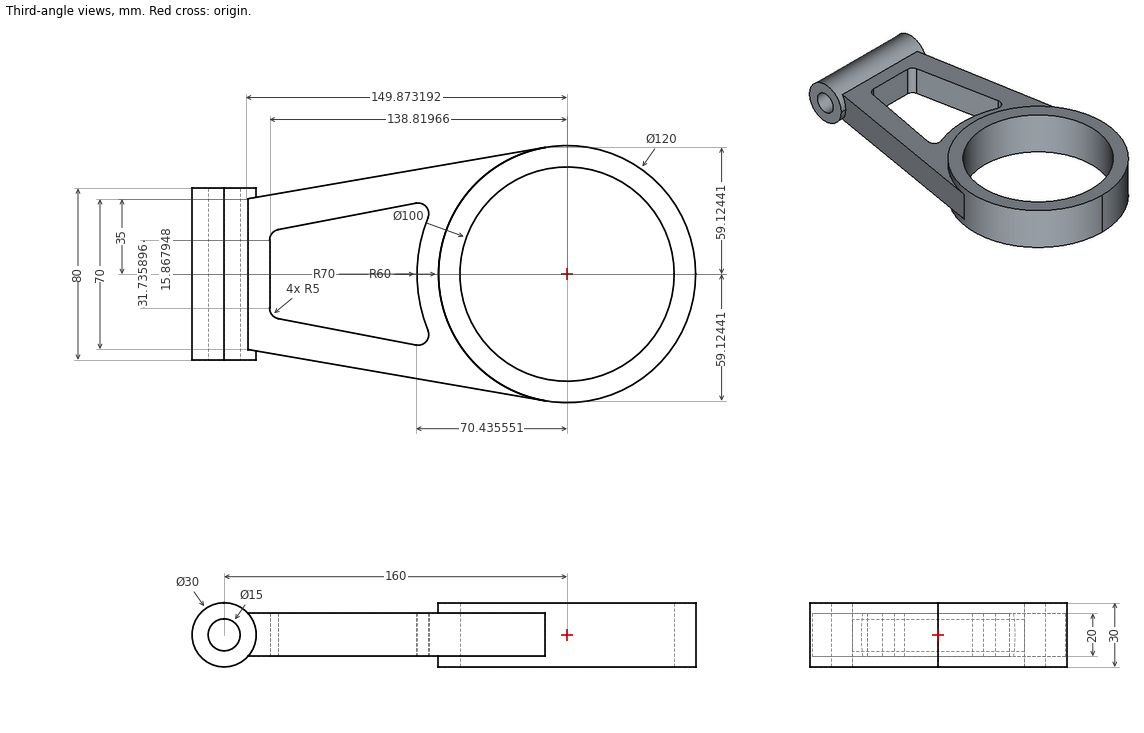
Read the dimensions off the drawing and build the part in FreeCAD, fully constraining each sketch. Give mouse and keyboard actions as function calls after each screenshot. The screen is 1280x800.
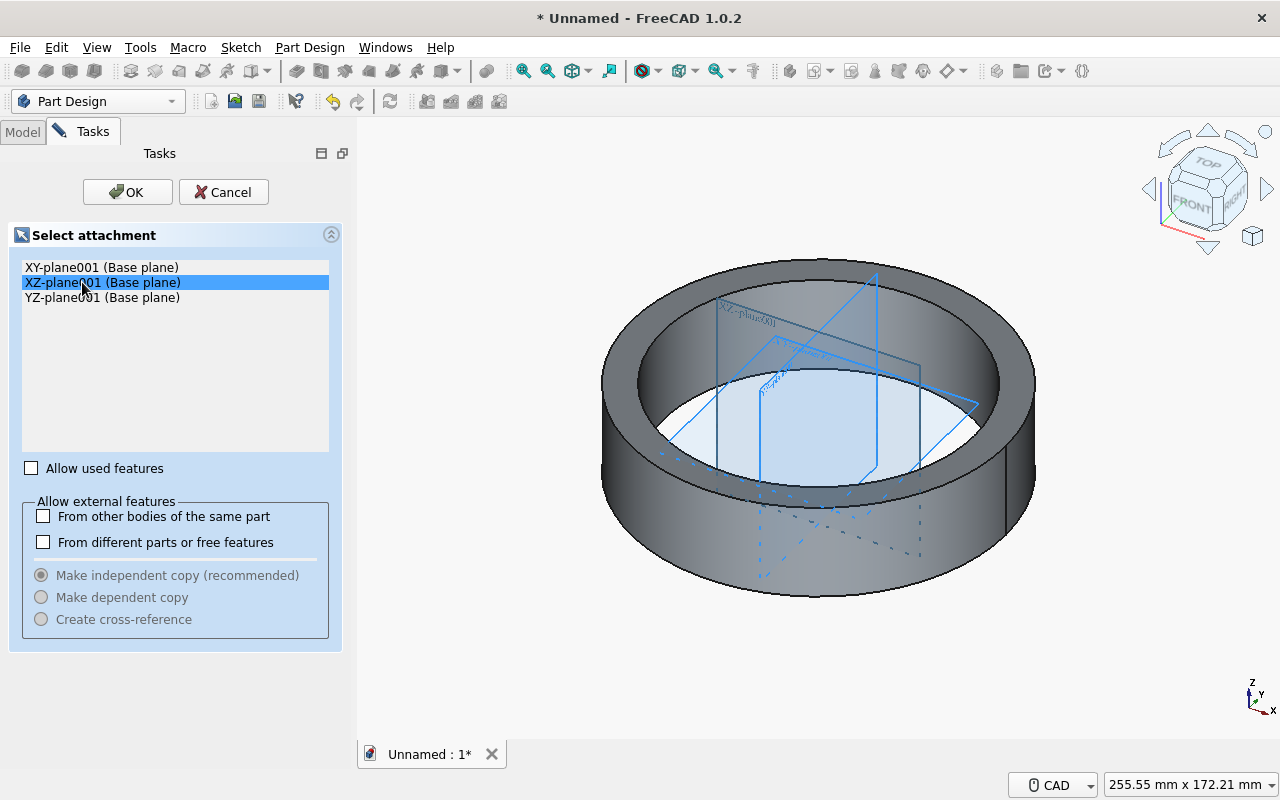
click(128, 192)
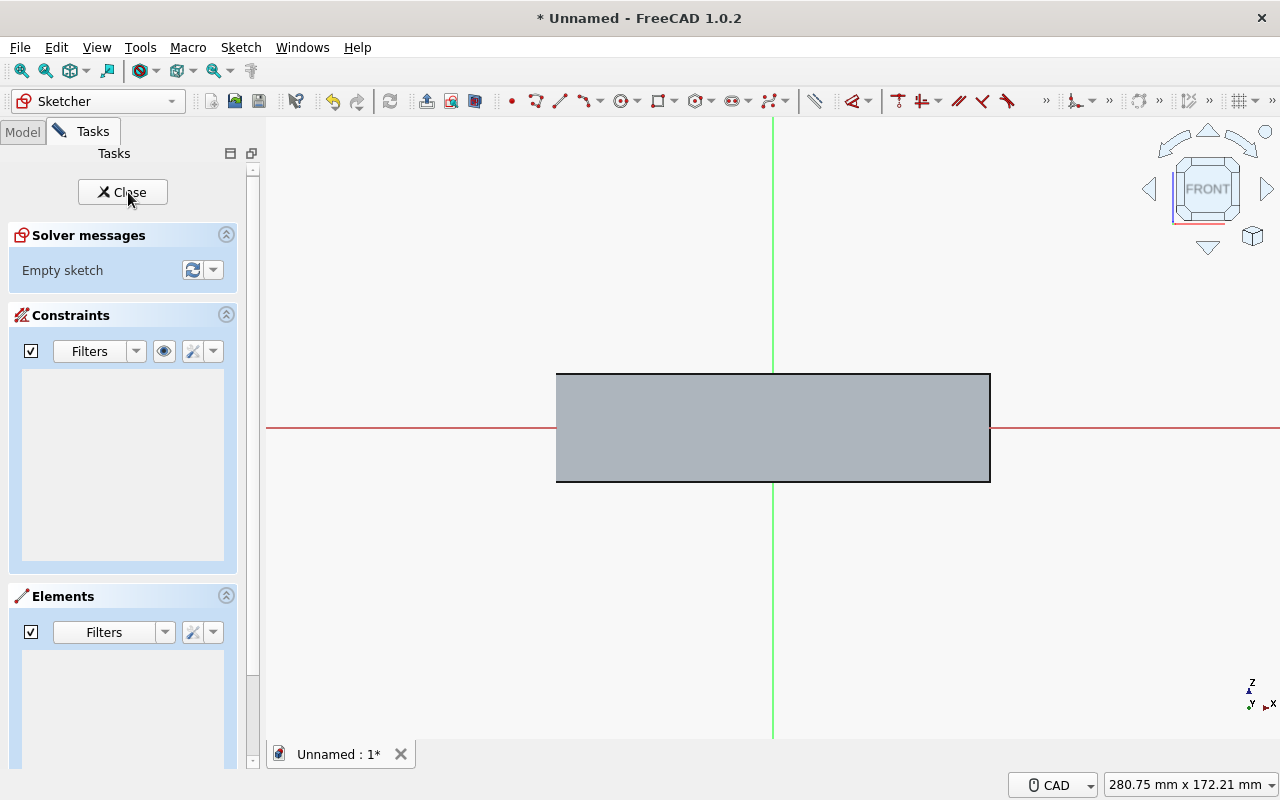
scroll(704, 428, down, 5)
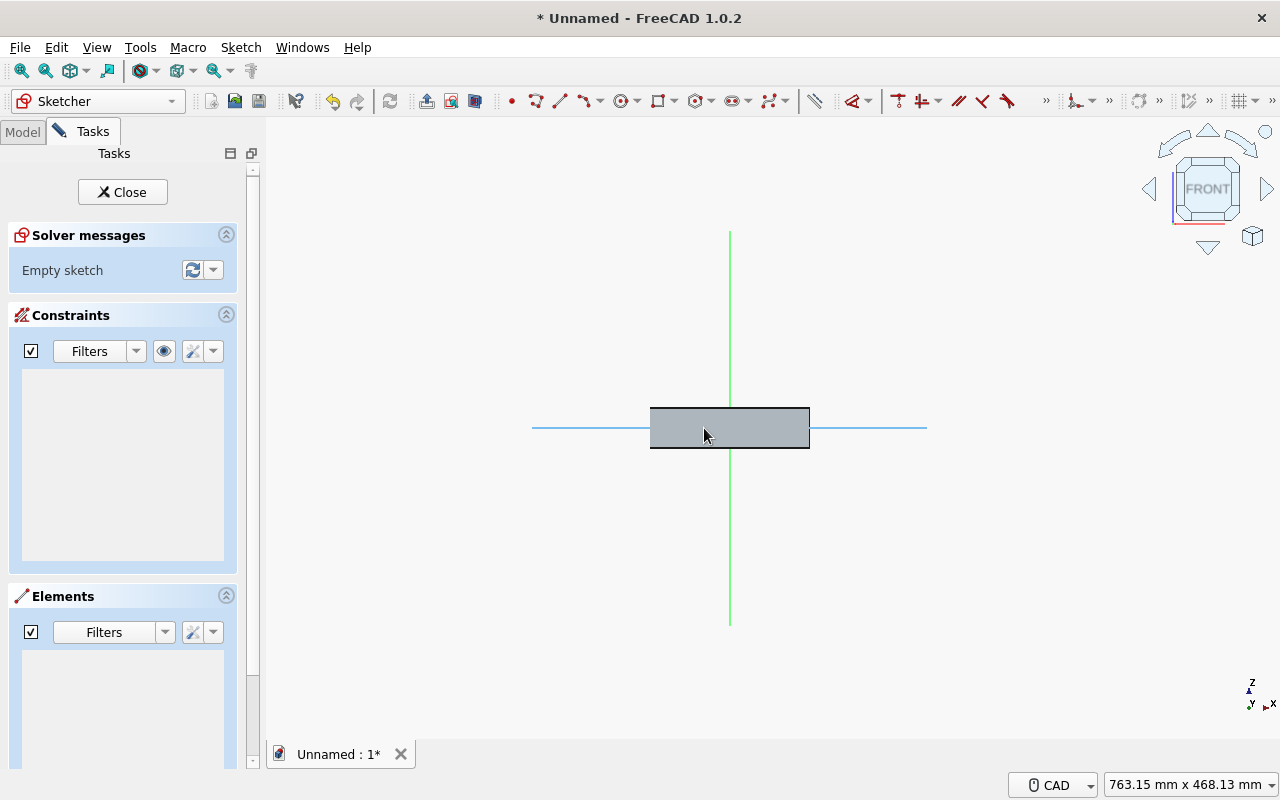
scroll(498, 428, up, 12)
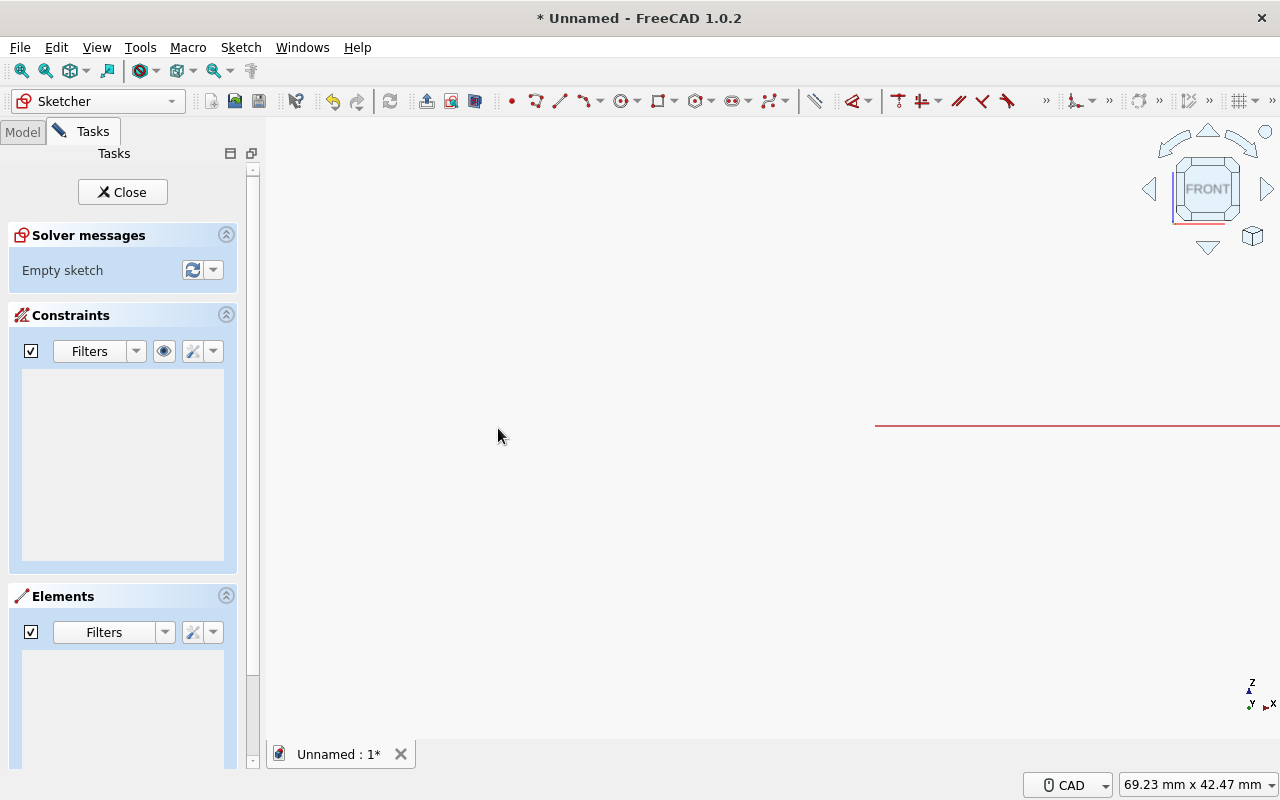
click(622, 102)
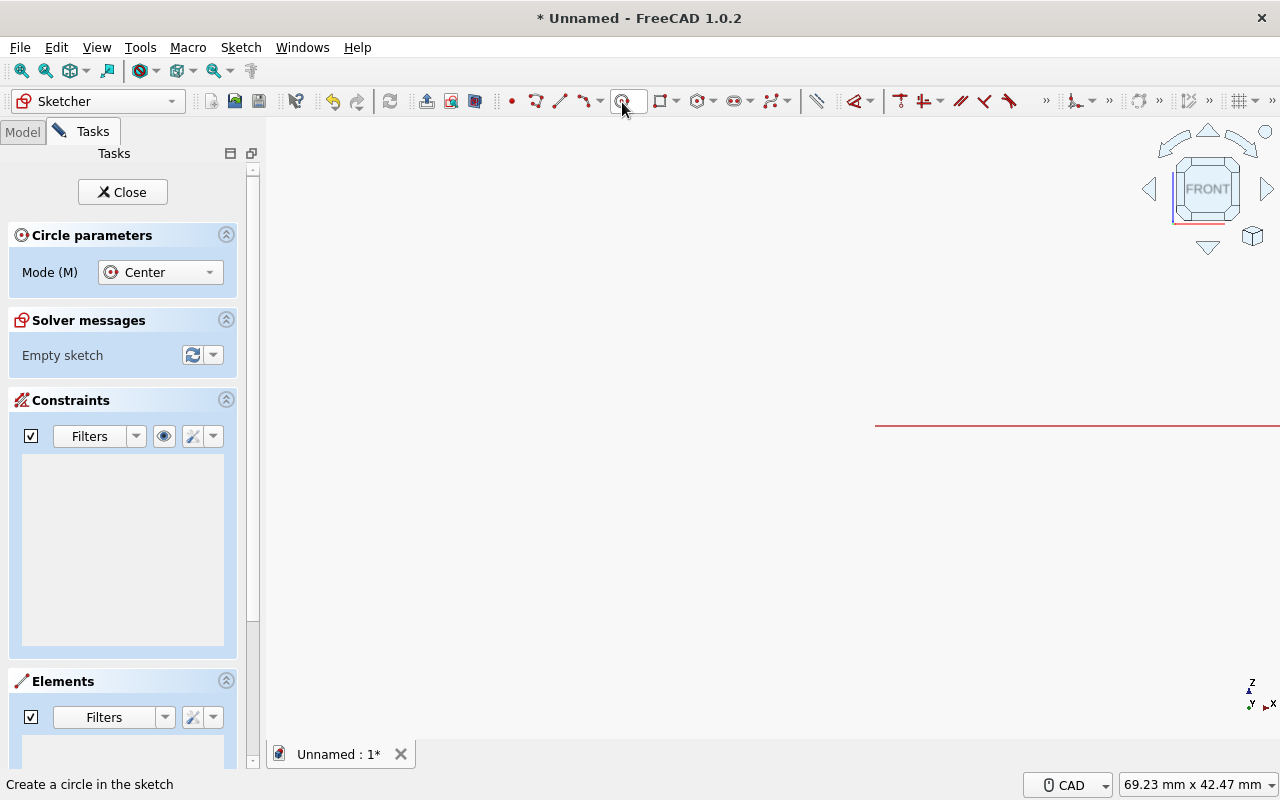
click(706, 426)
move(861, 271)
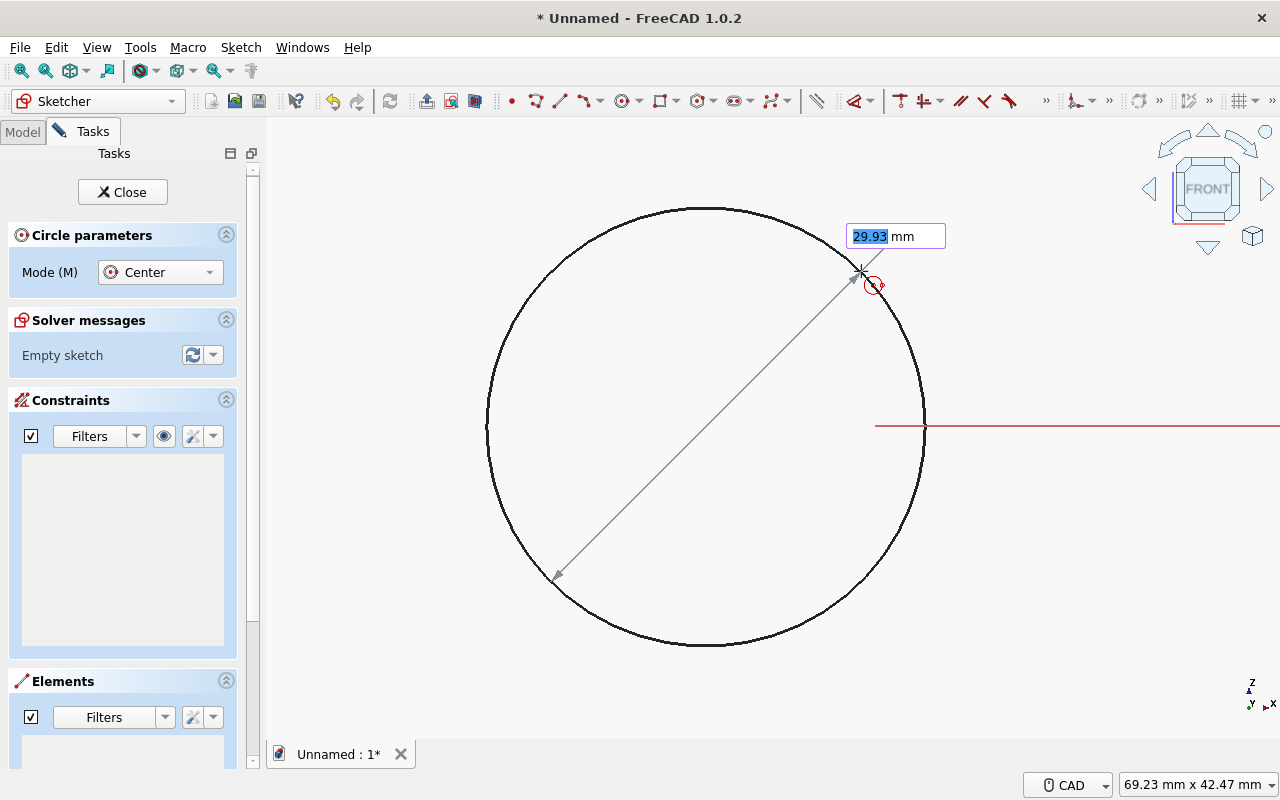
text(30)
key(Return)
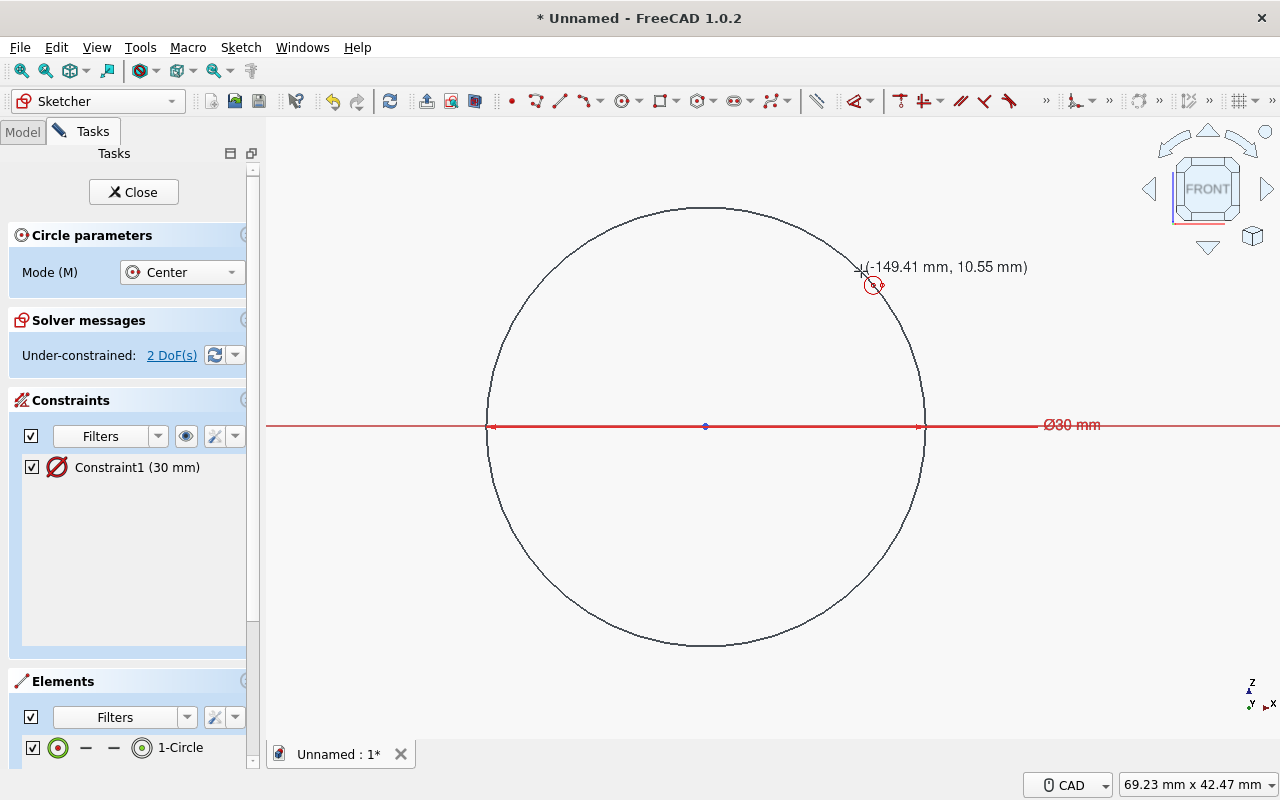
click(706, 427)
move(784, 349)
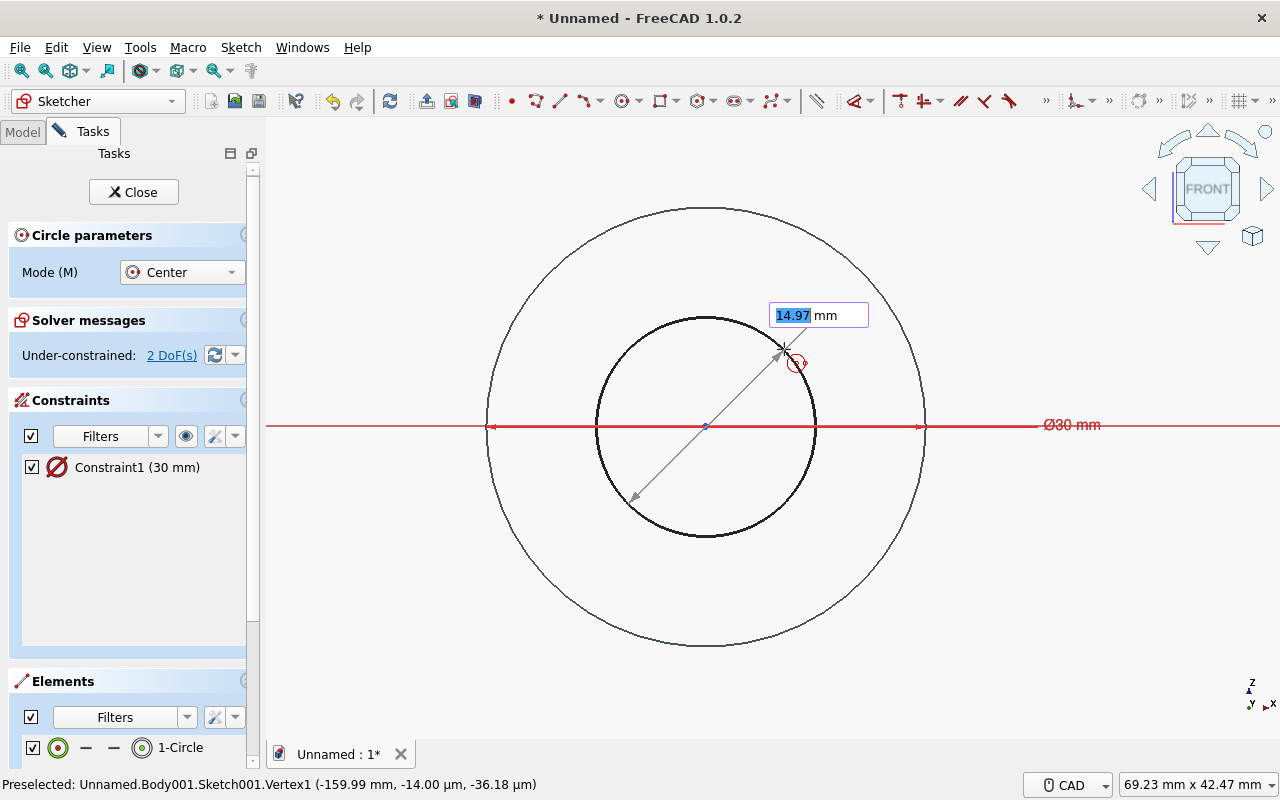
text(15)
key(Return)
key(Escape)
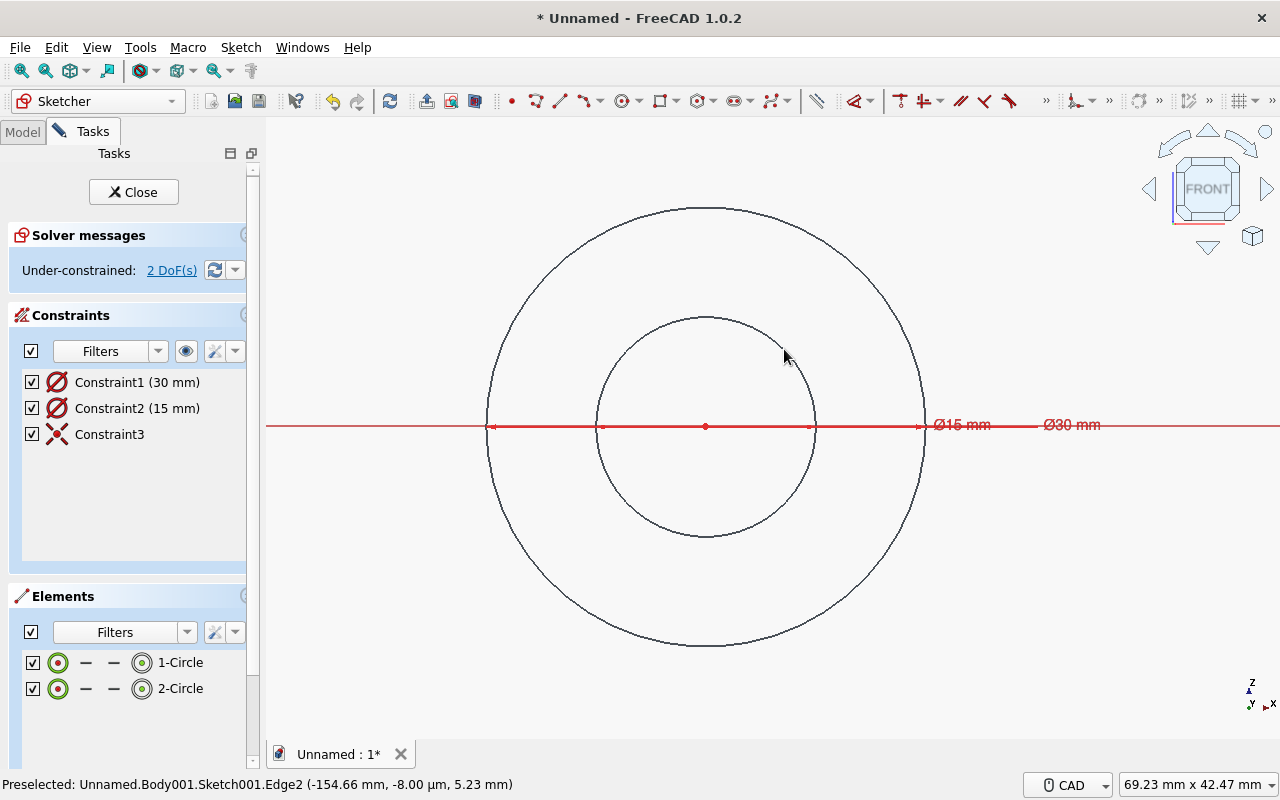
click(706, 427)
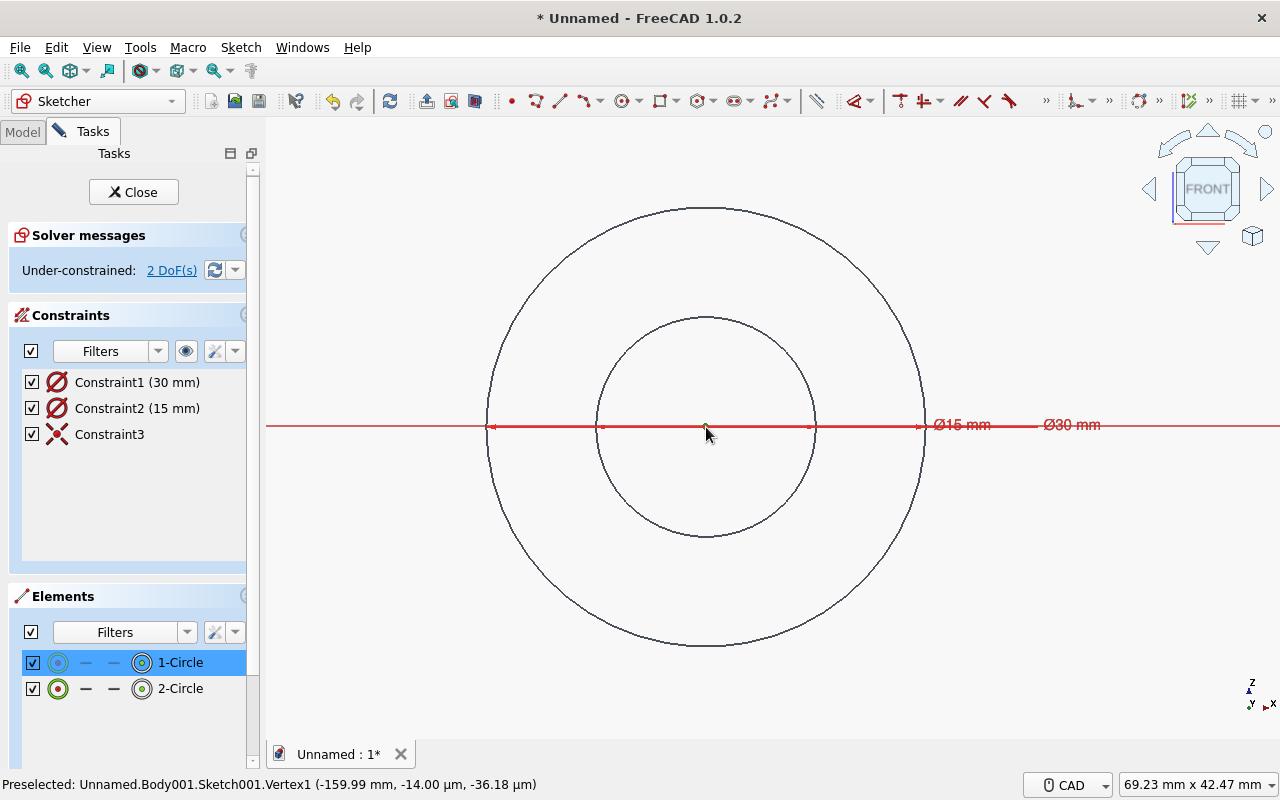
click(353, 426)